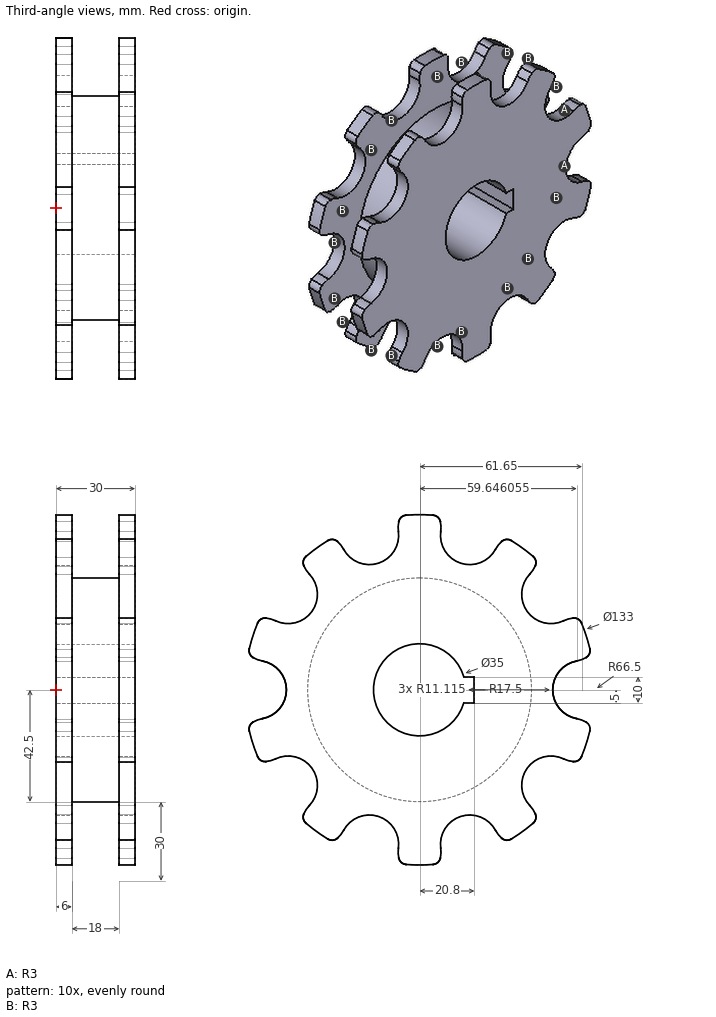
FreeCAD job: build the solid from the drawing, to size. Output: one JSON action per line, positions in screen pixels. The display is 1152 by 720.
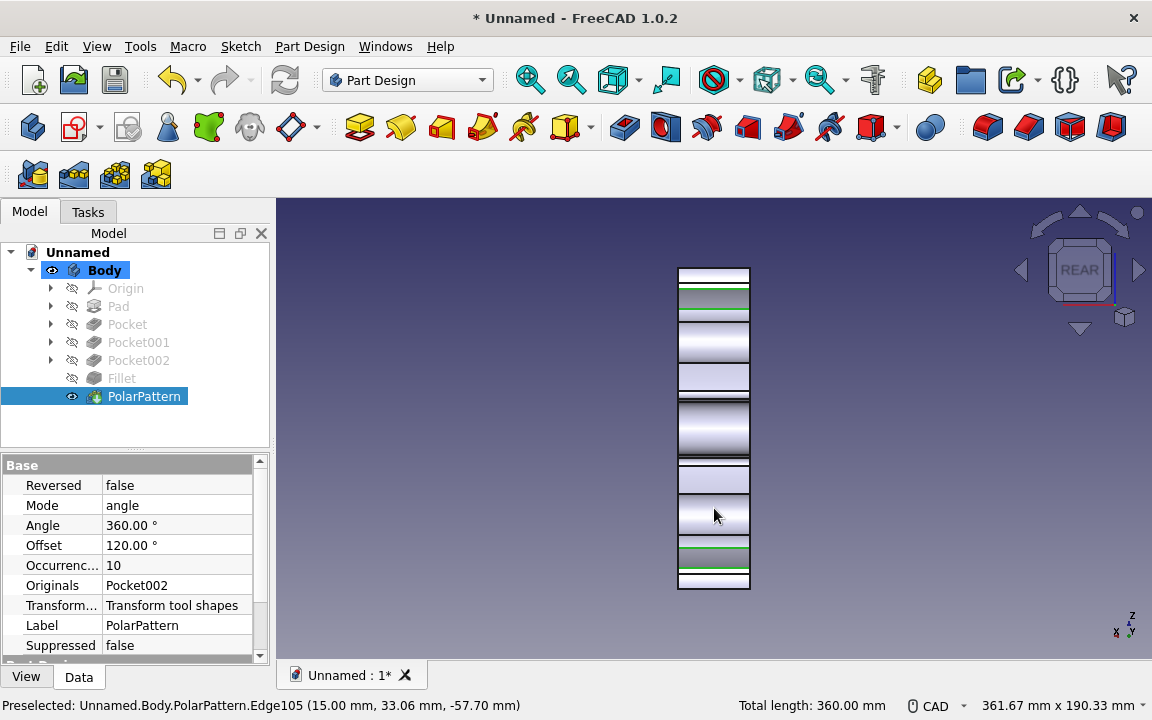
{"action": "key", "text": "6"}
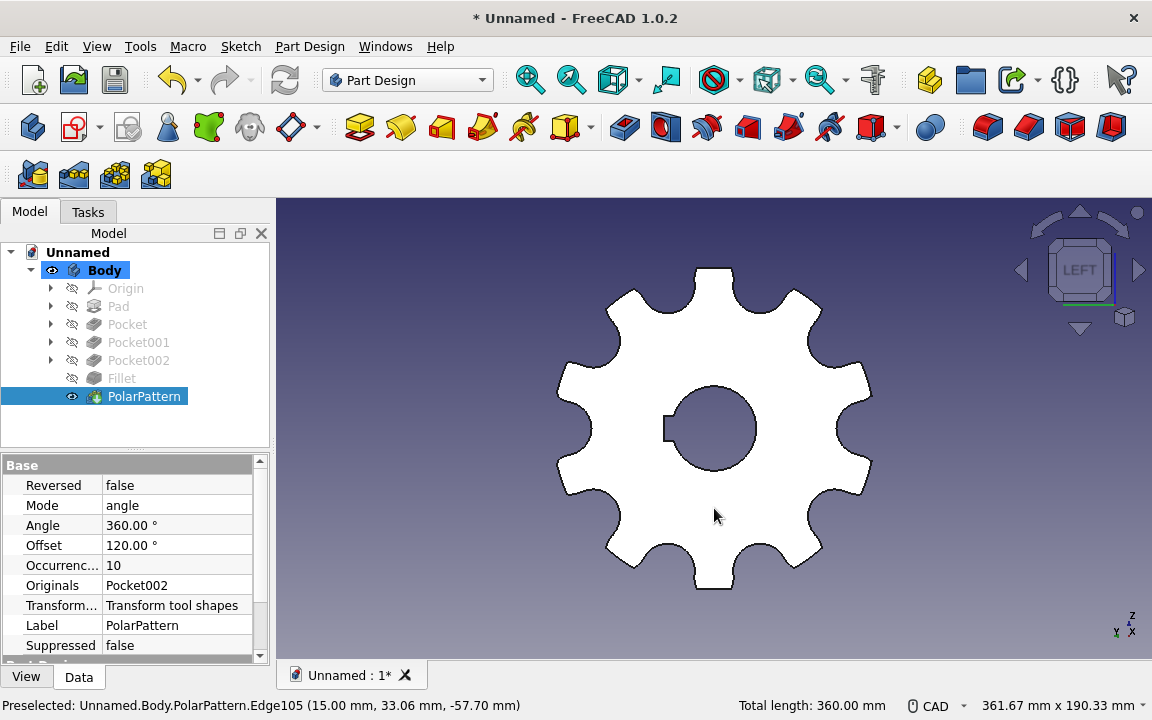
{"action": "key", "text": "v 3"}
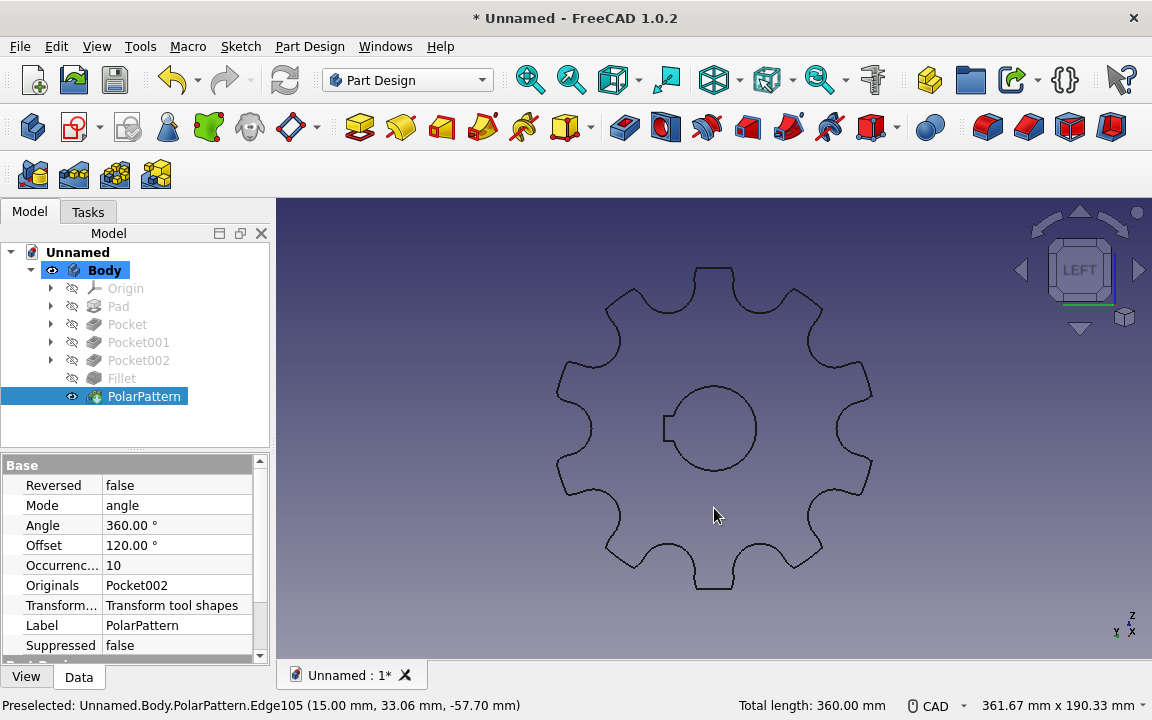
{"action": "key", "text": "0"}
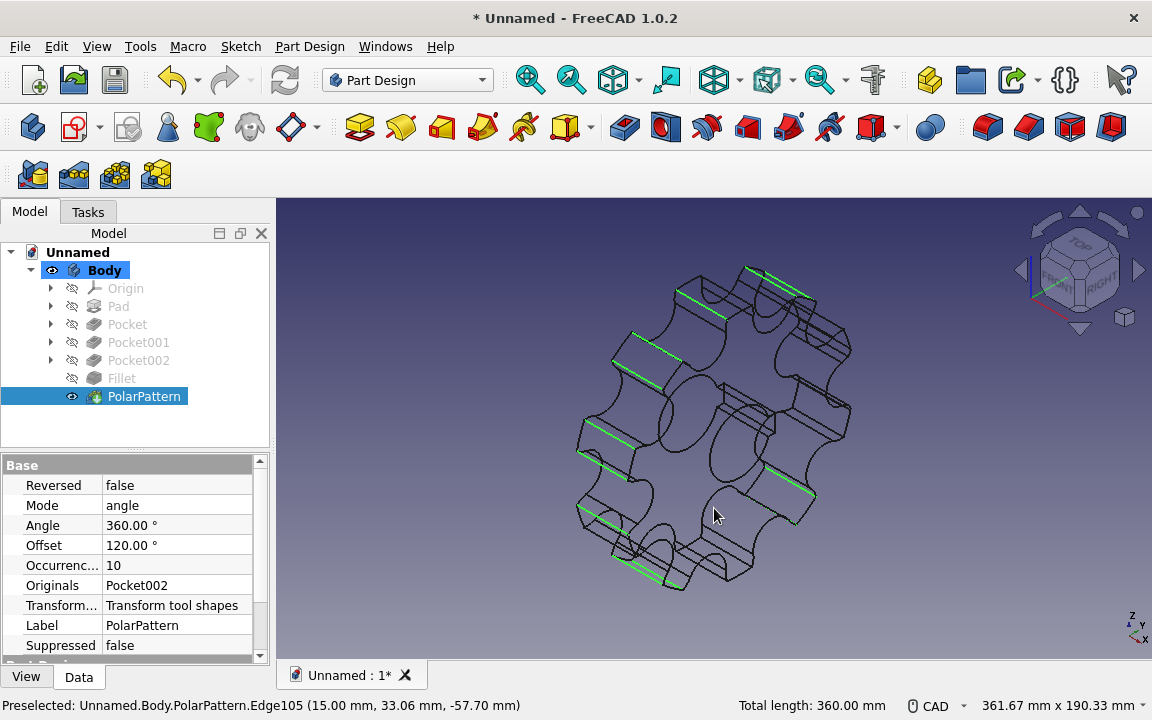
{"action": "left_click", "coordinate": [823, 317], "text": "ctrl"}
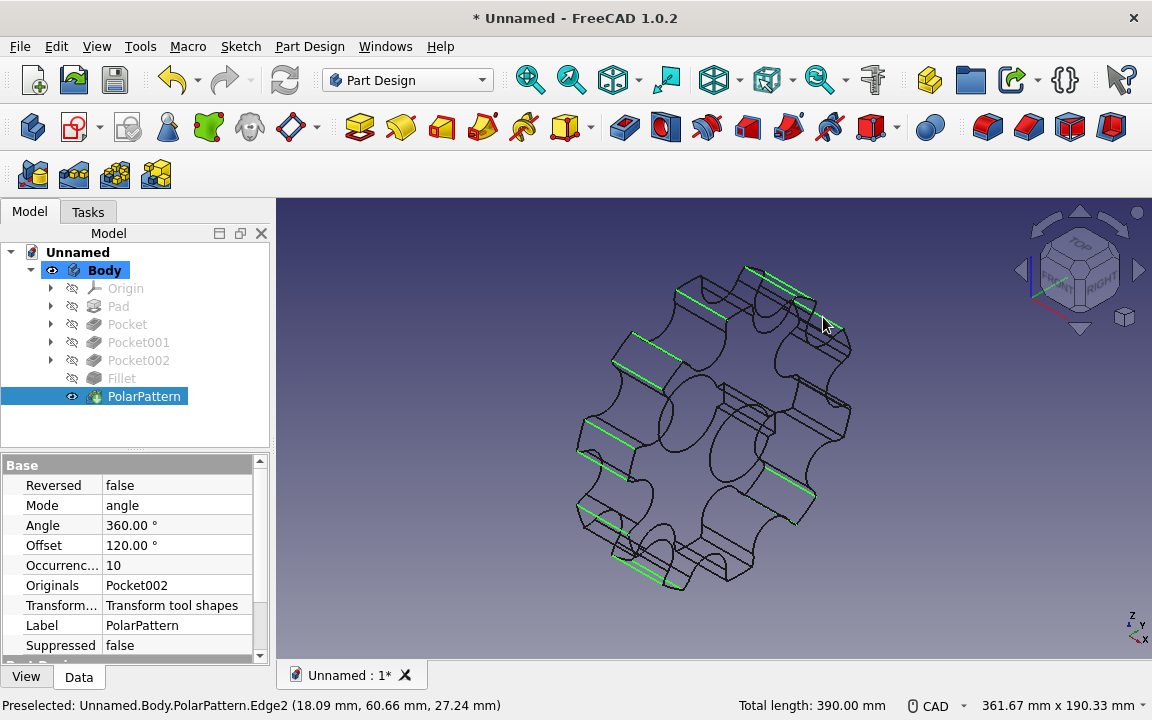
{"action": "left_click", "coordinate": [726, 290], "text": "ctrl"}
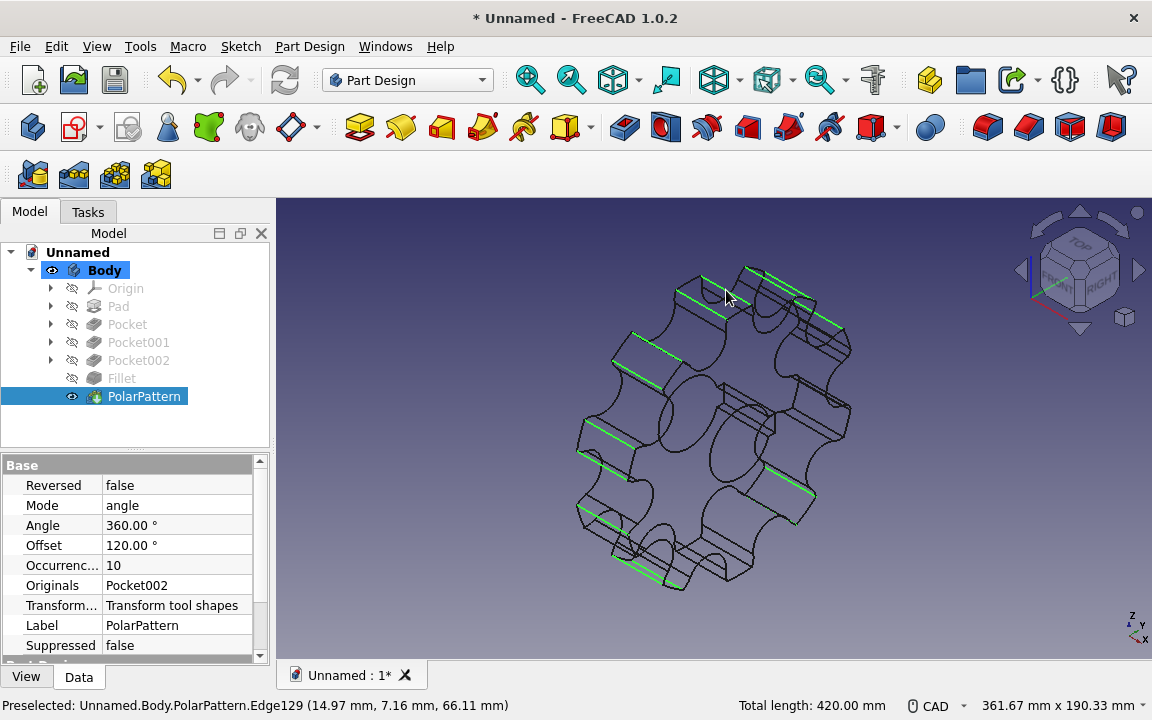
{"action": "left_click", "coordinate": [610, 541], "text": "ctrl"}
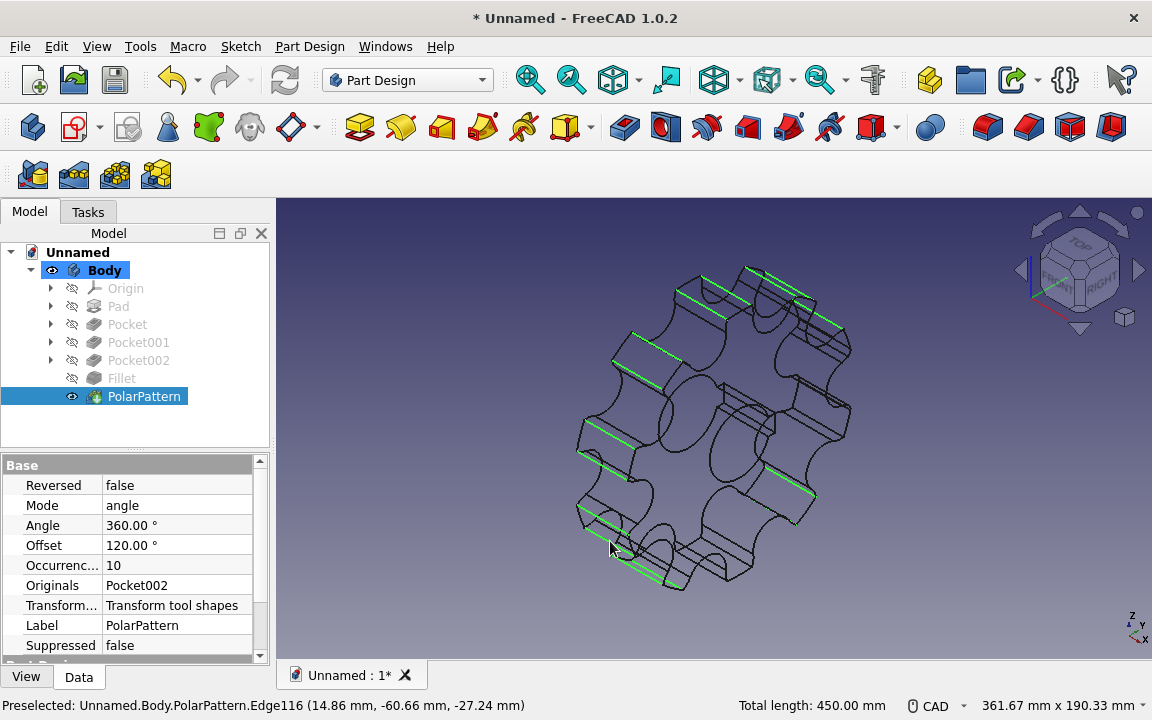
{"action": "left_click", "coordinate": [707, 568], "text": "ctrl"}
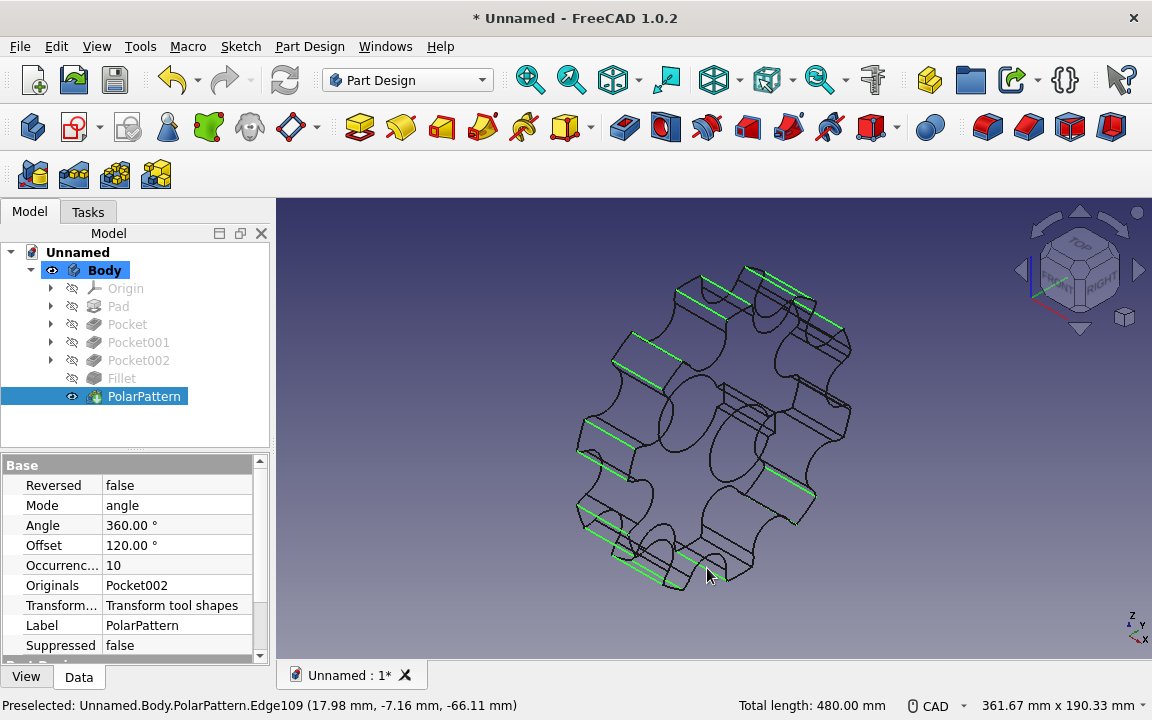
{"action": "left_click", "coordinate": [731, 554], "text": "ctrl"}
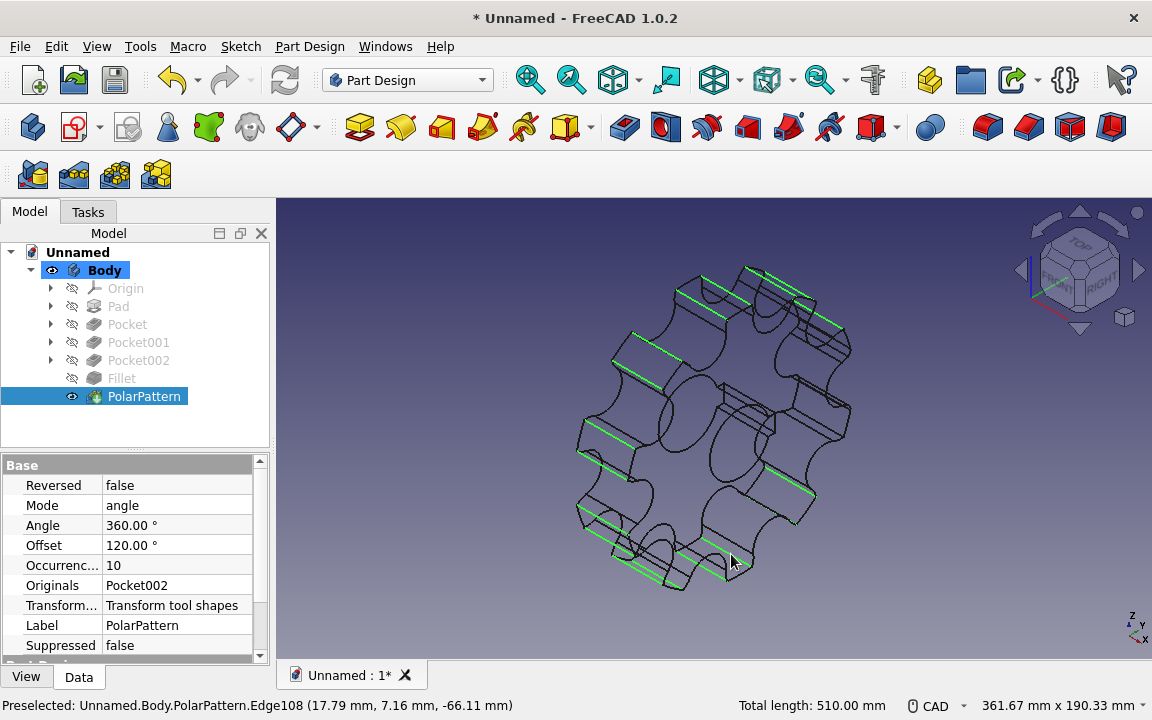
{"action": "left_click", "coordinate": [818, 421], "text": "ctrl"}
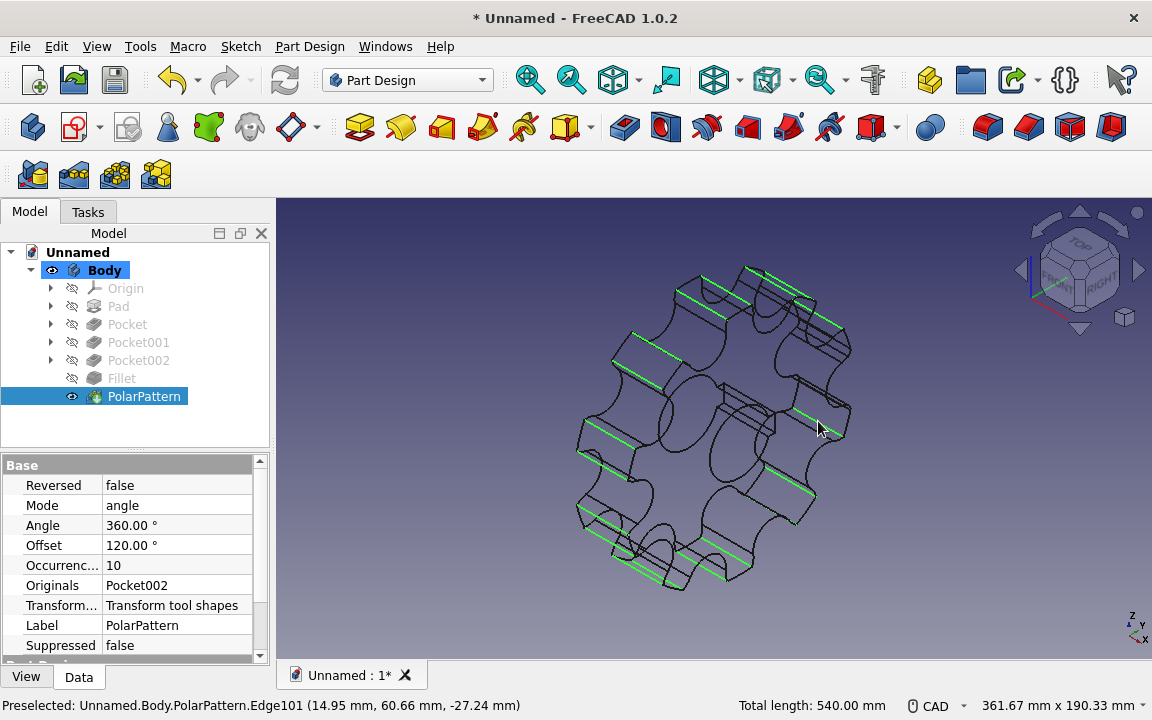
{"action": "key", "text": "v 1"}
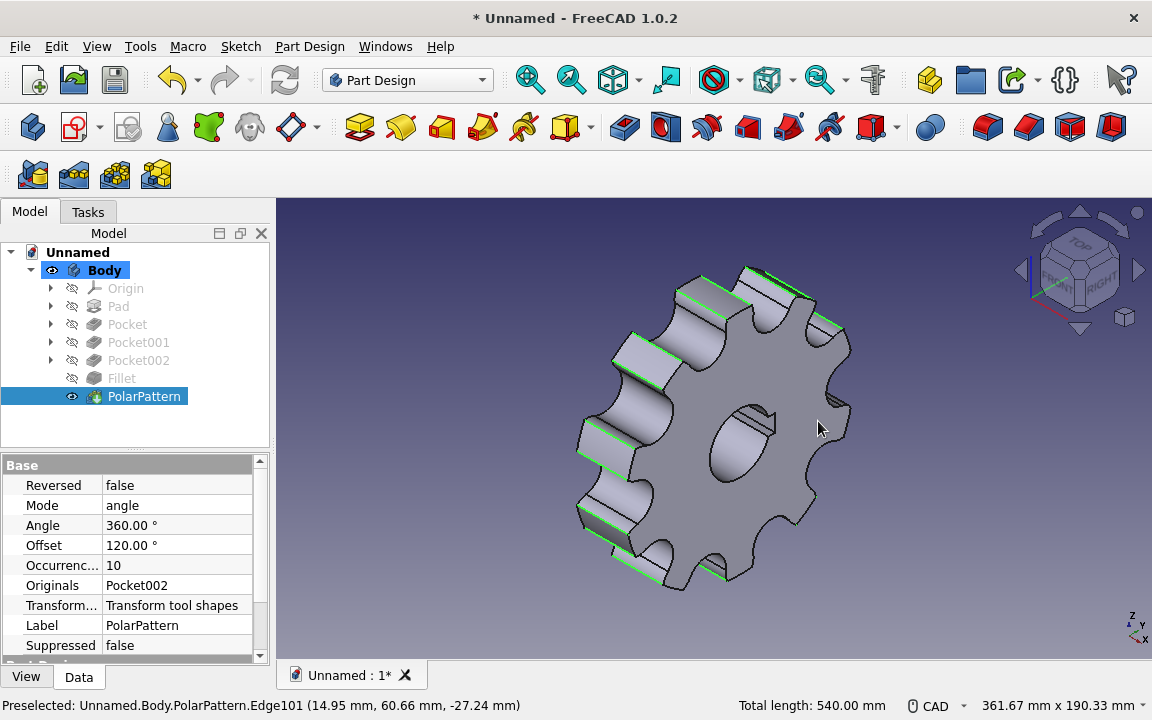
{"action": "left_click", "coordinate": [988, 128]}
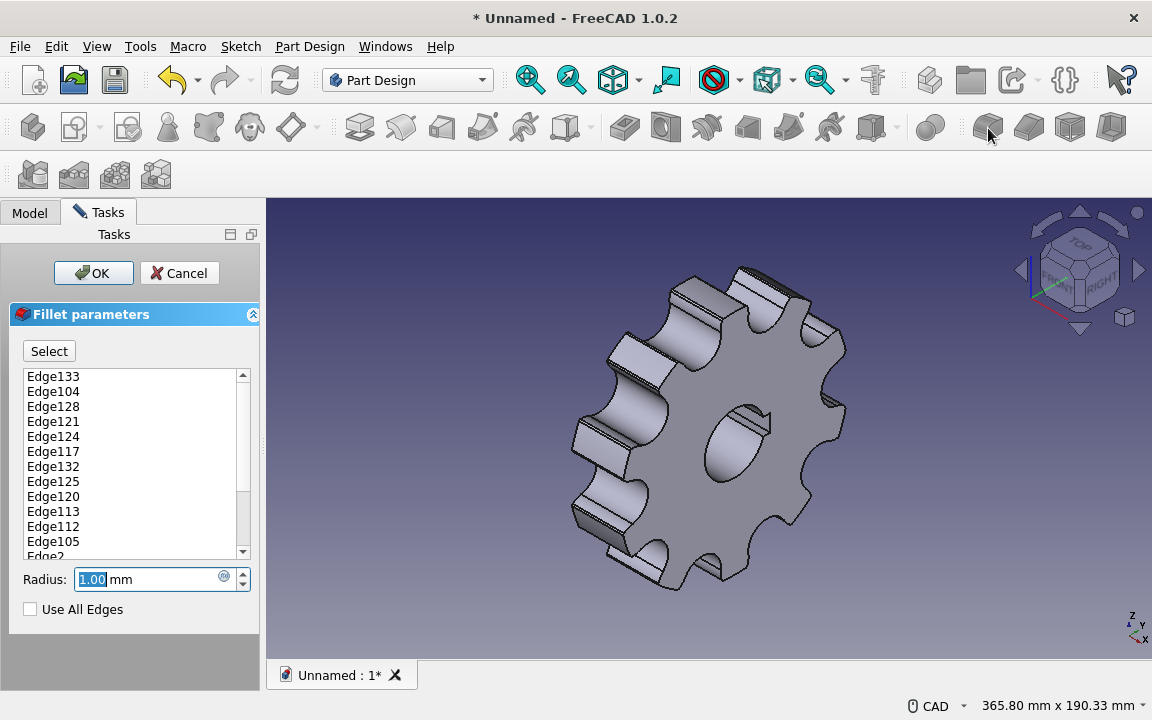
{"action": "type", "text": "3"}
{"action": "key", "text": "Tab"}